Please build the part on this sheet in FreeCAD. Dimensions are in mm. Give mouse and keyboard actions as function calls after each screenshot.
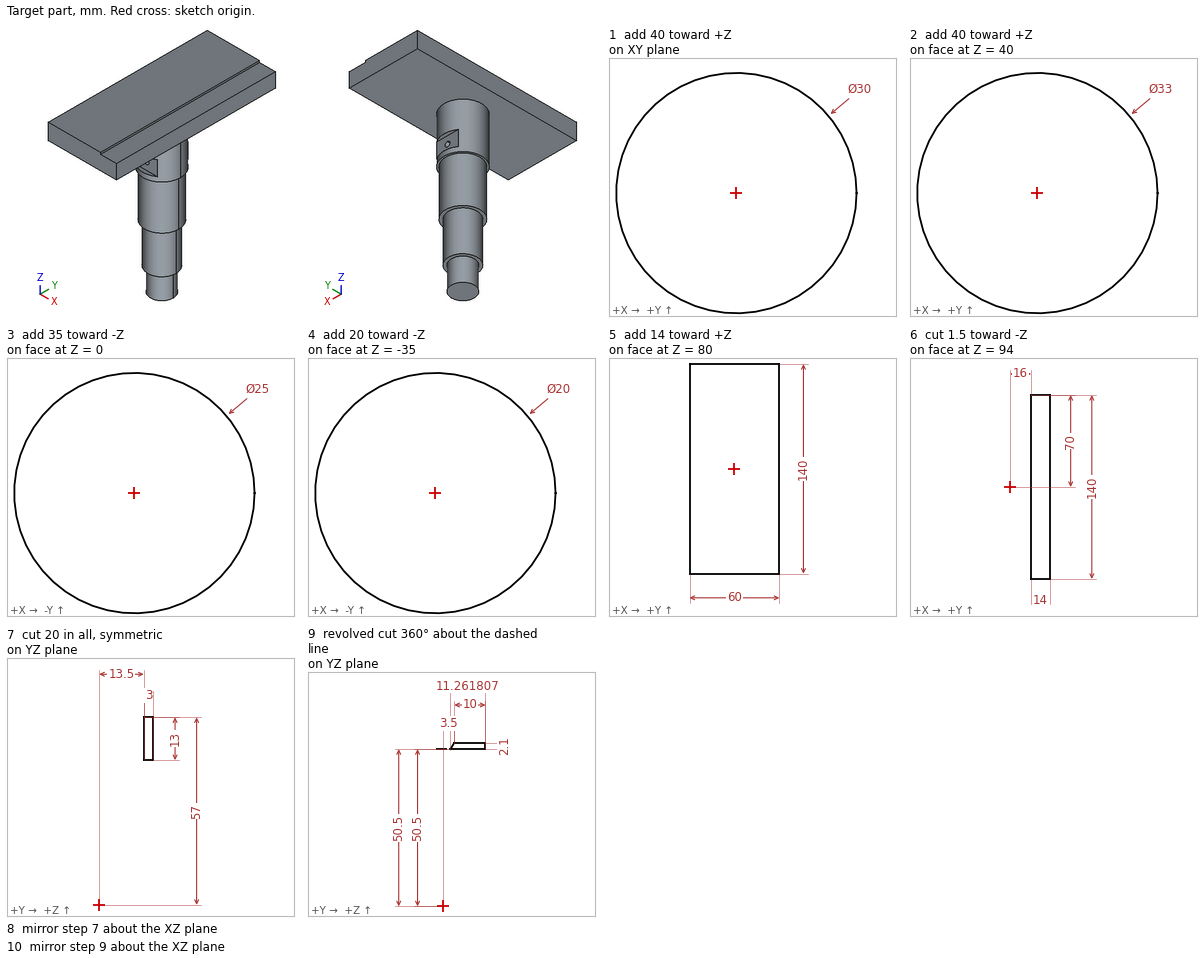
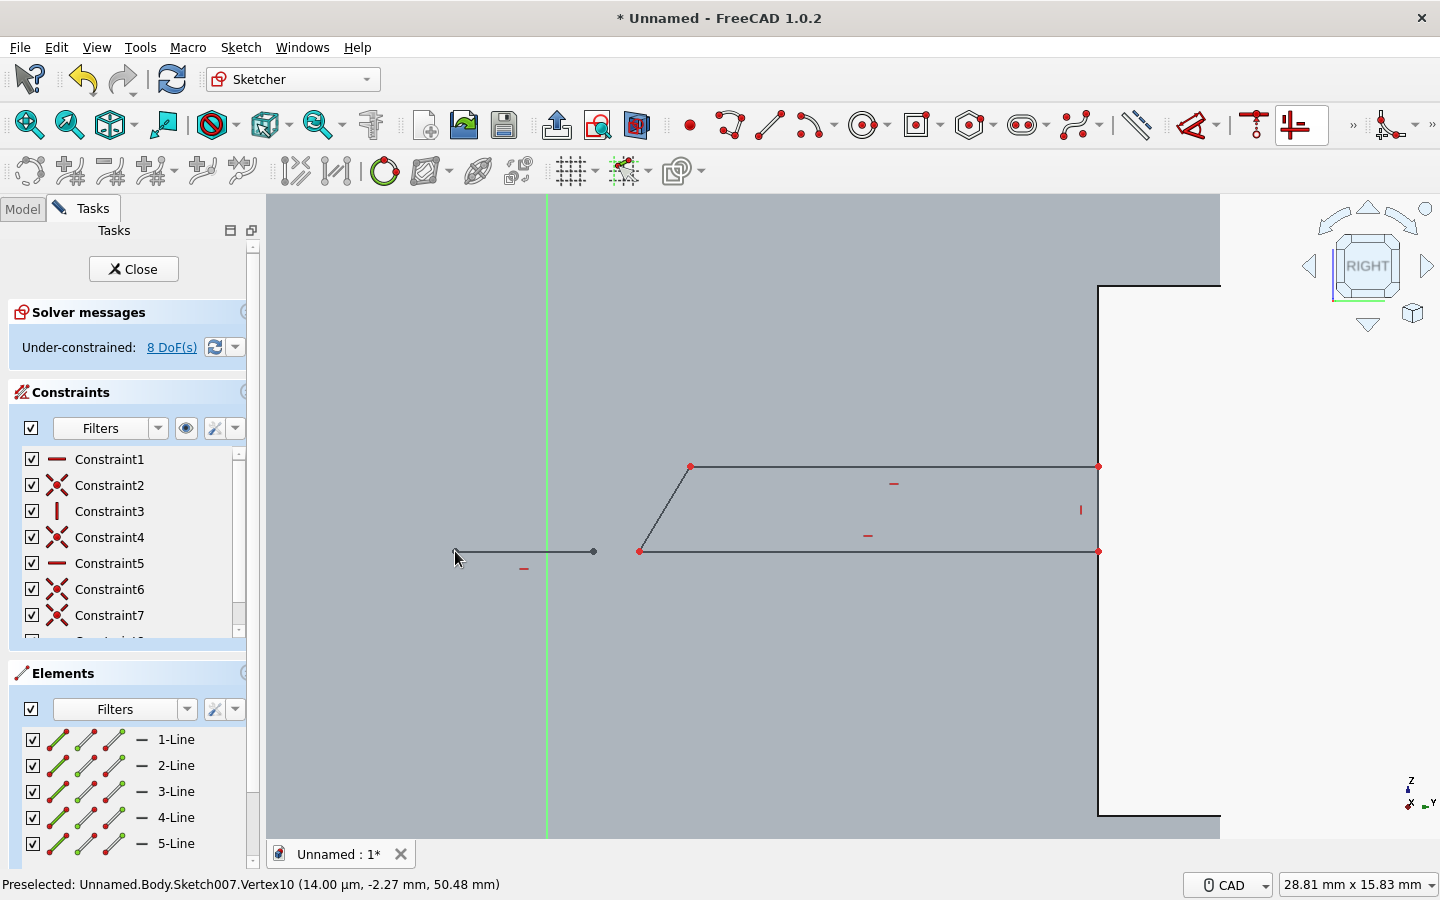
click(496, 552)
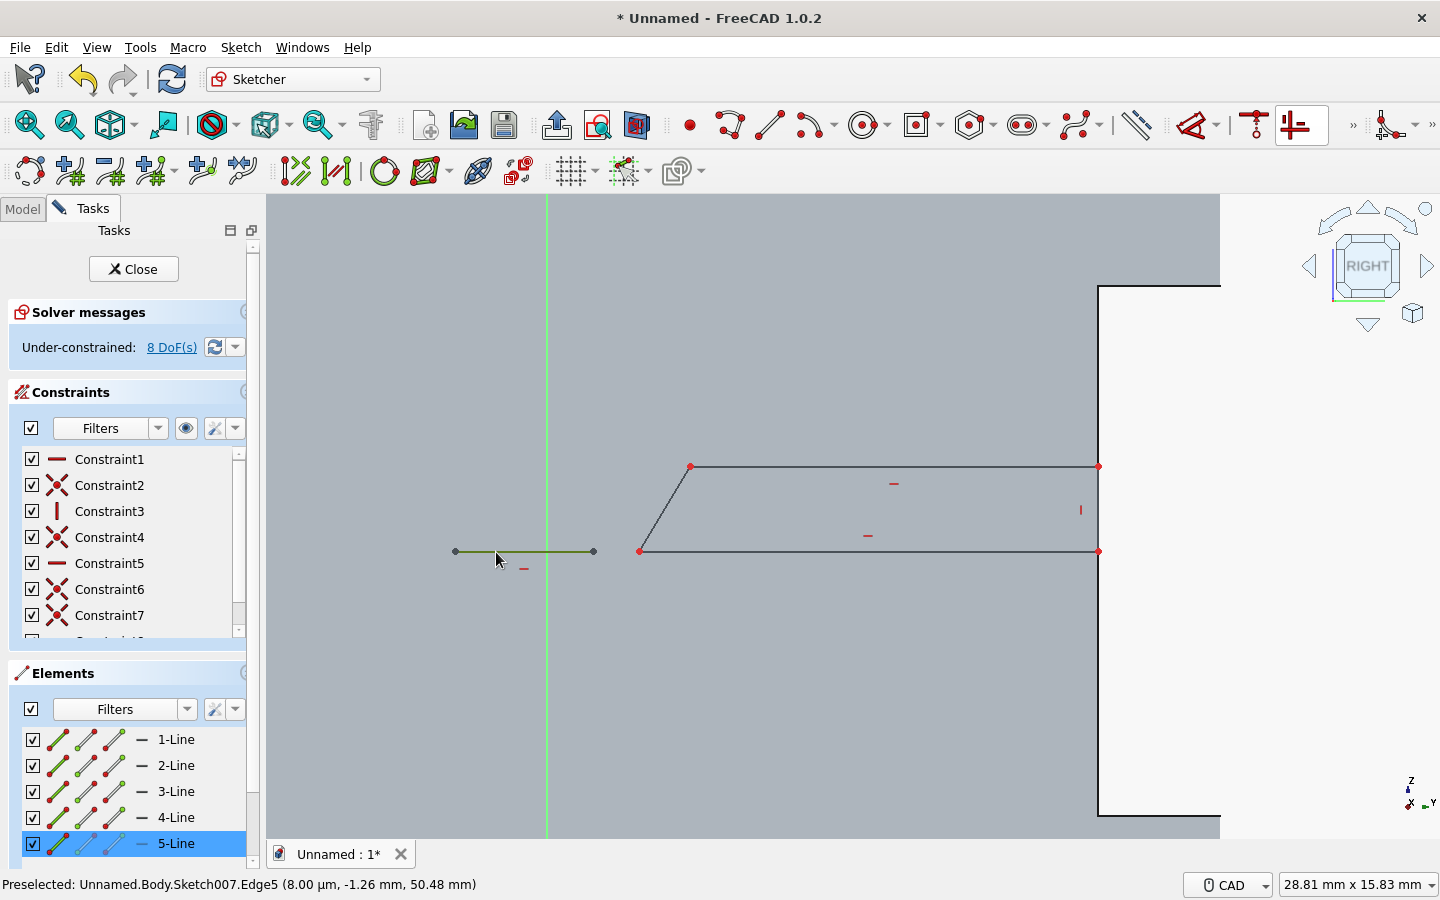
click(1138, 126)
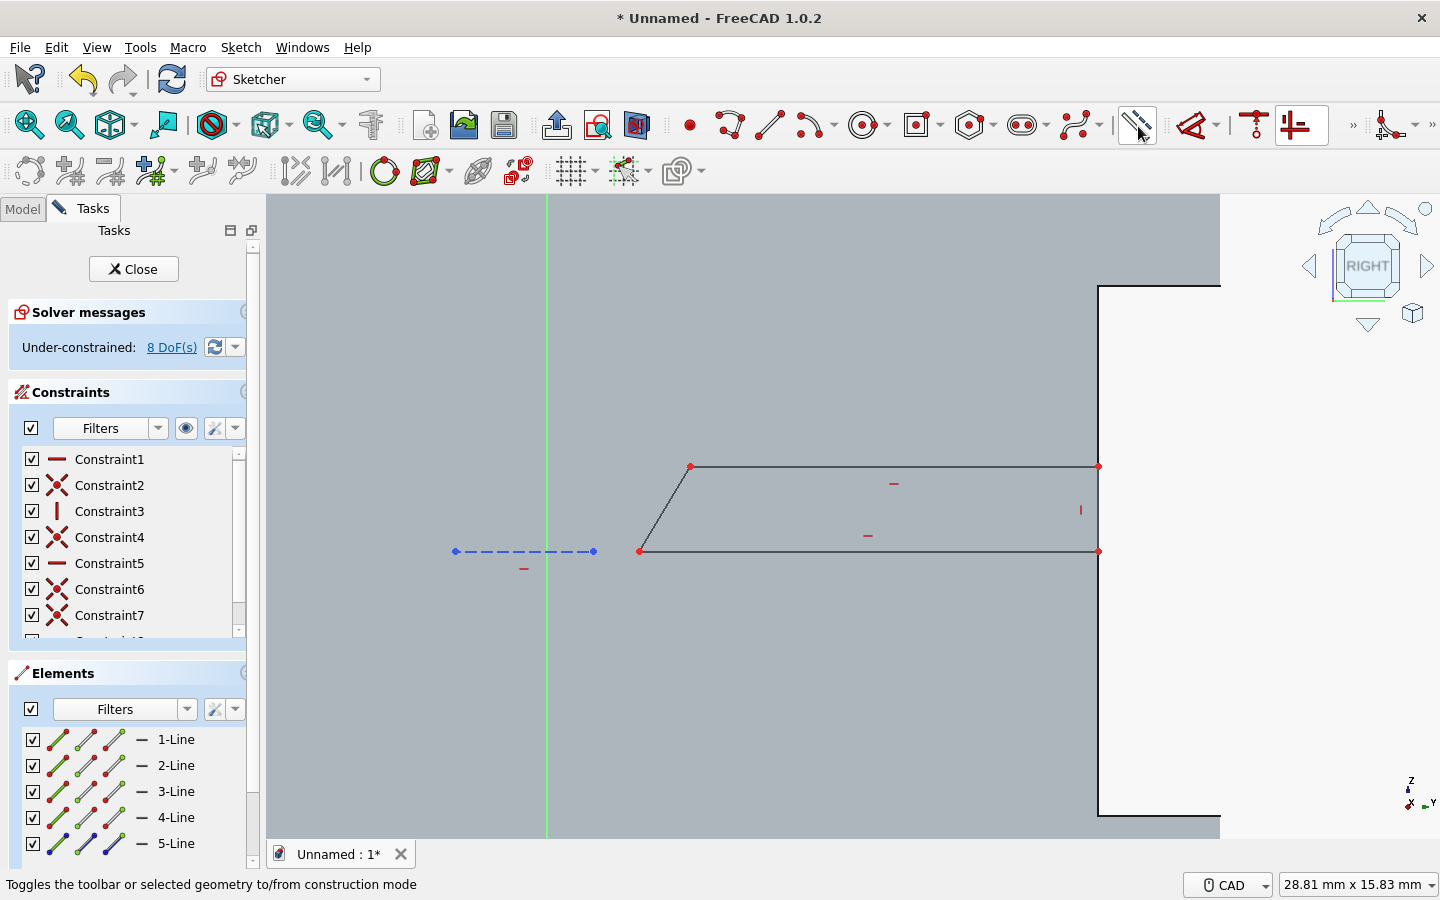
click(1192, 126)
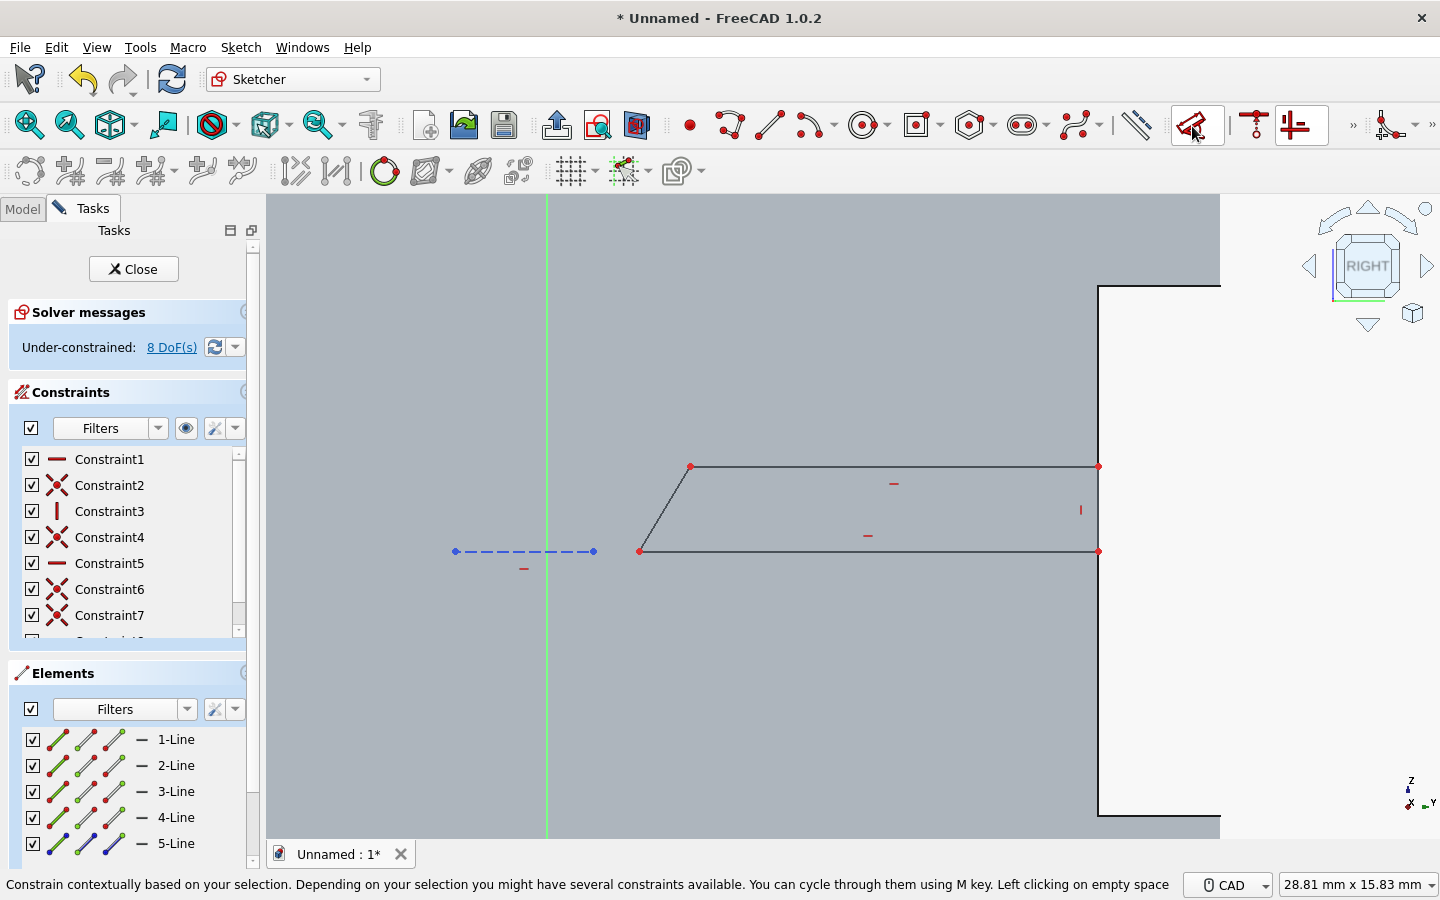
click(976, 467)
click(894, 433)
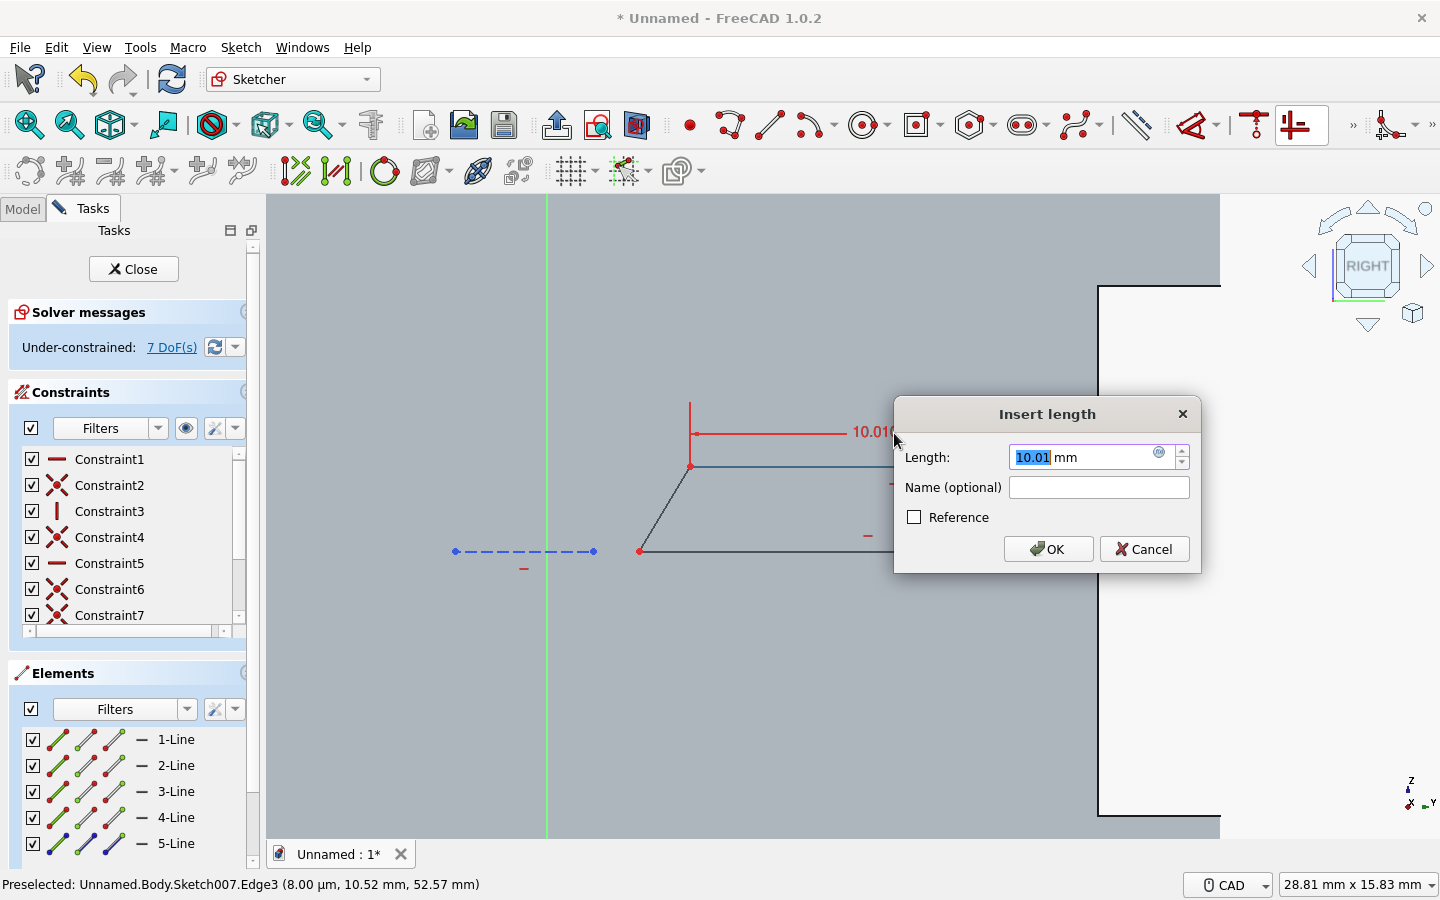
text(10)
key(Return)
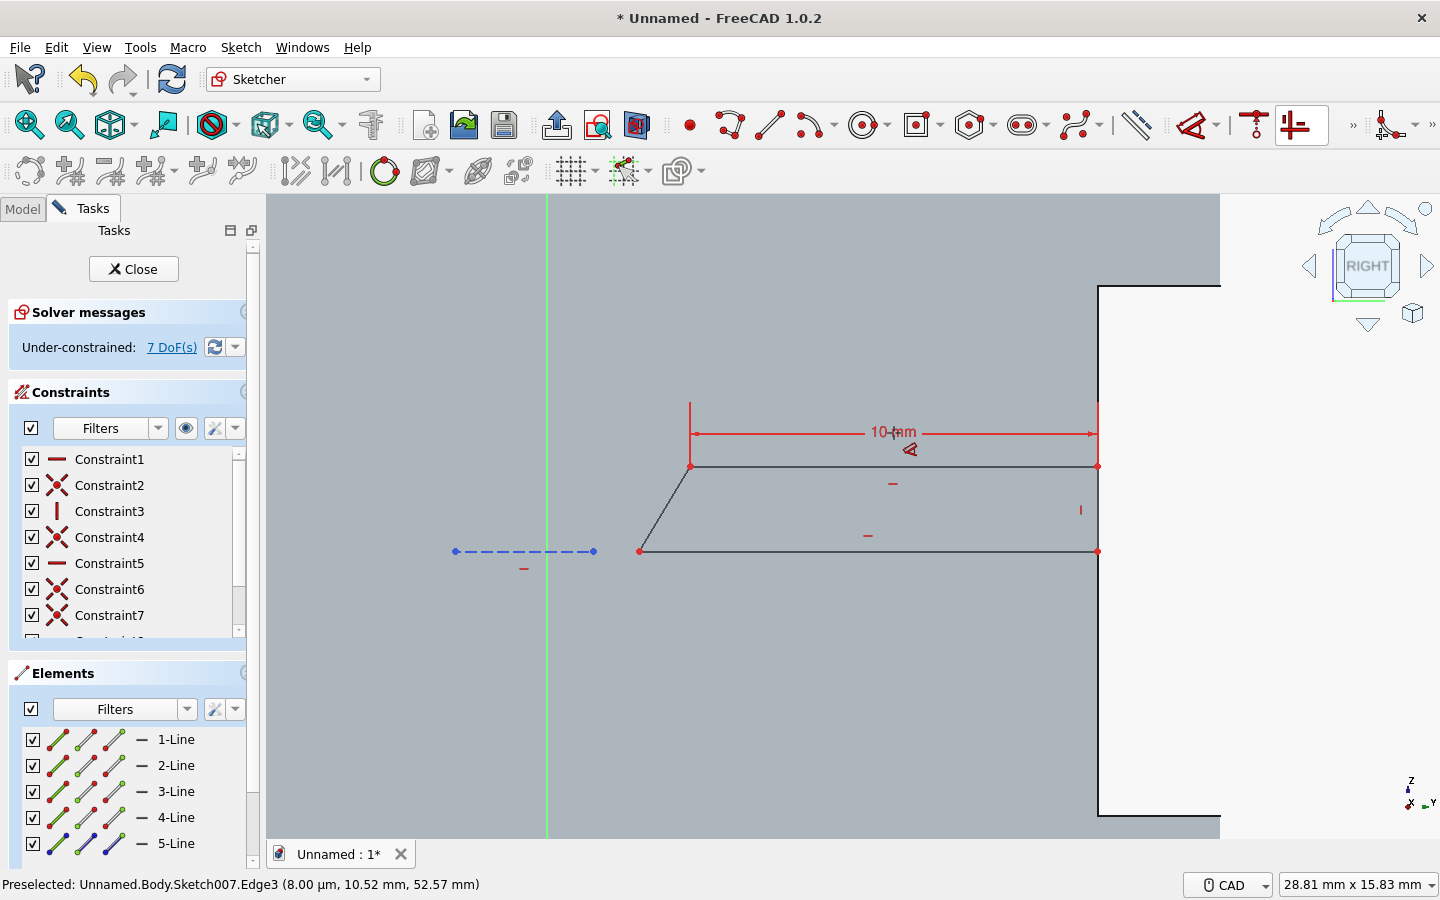
click(1098, 527)
click(1132, 510)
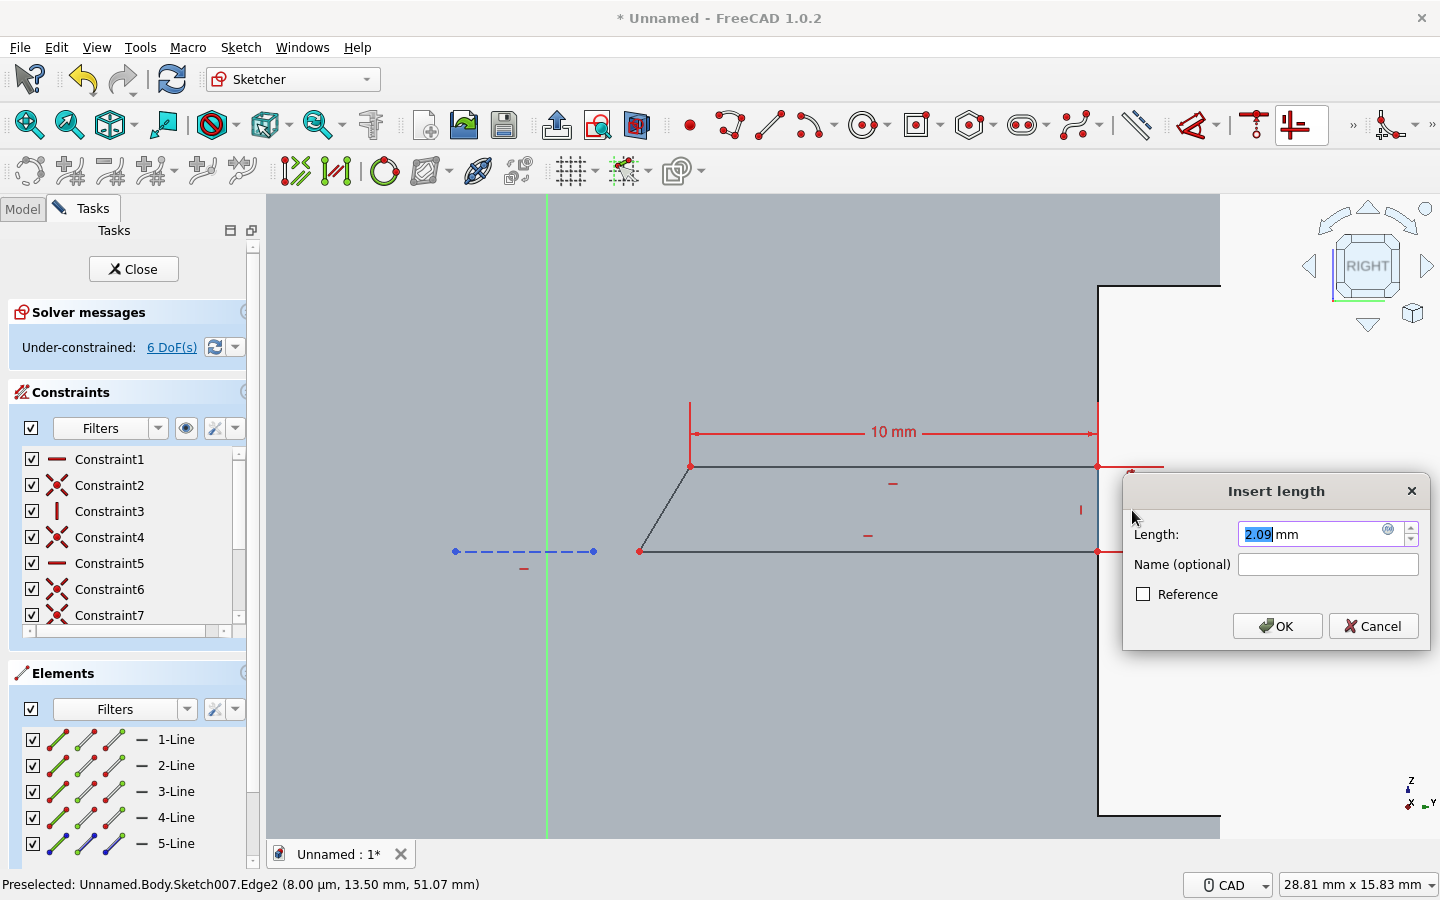
text(2.1)
key(Return)